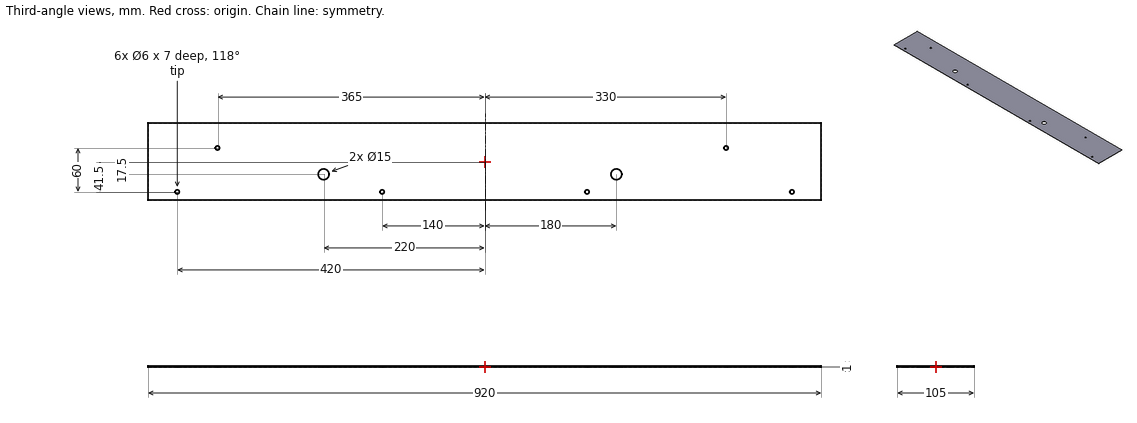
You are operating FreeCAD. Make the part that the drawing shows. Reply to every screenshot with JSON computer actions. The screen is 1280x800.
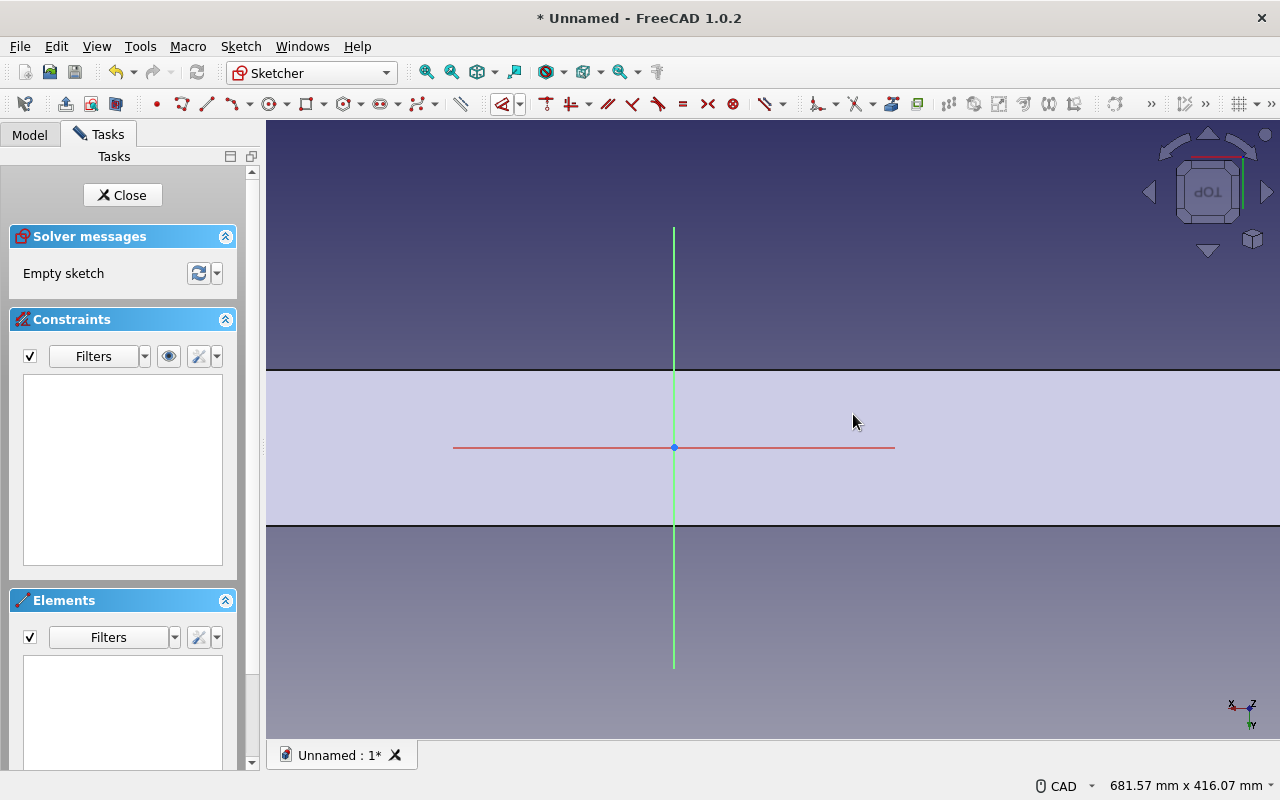
{"action": "left_click", "coordinate": [268, 104]}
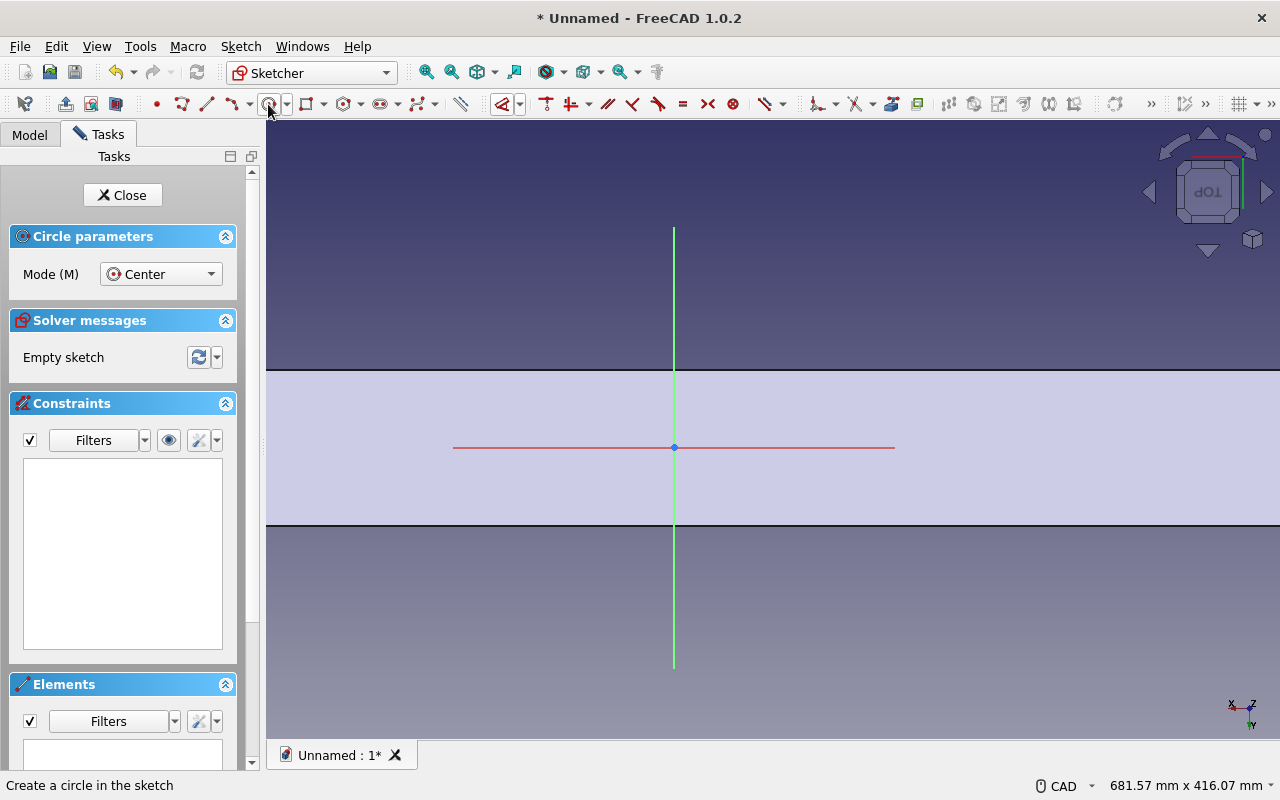
{"action": "scroll", "coordinate": [1002, 422], "scroll_direction": "up", "scroll_amount": 4}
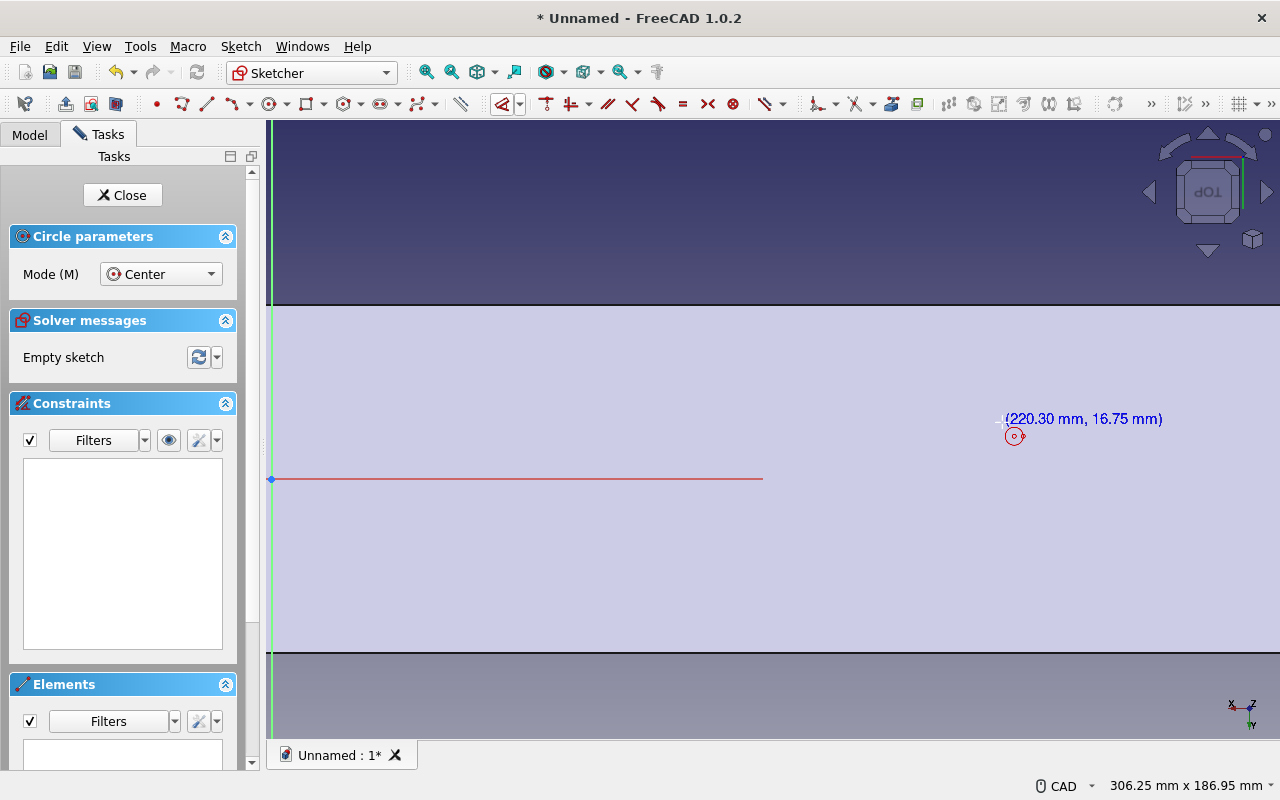
{"action": "left_click", "coordinate": [1000, 421]}
{"action": "left_click", "coordinate": [1018, 404]}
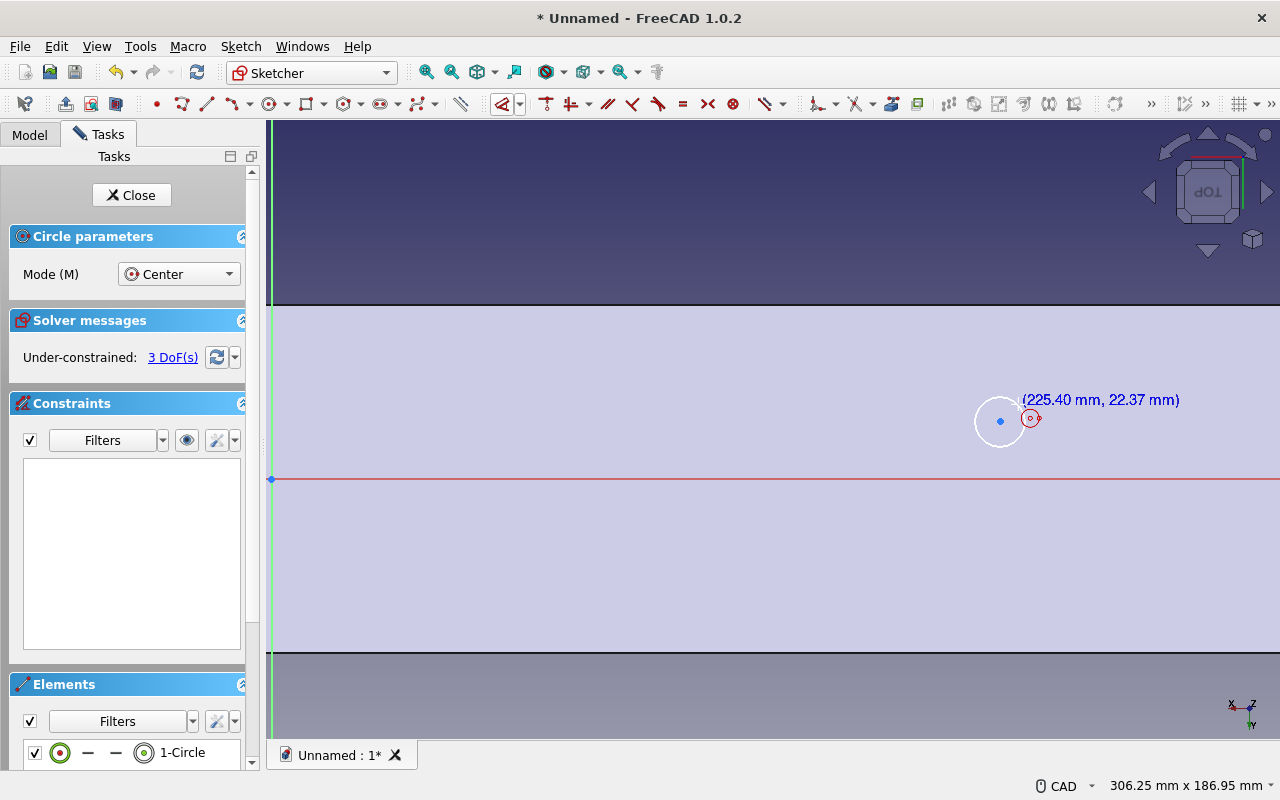
{"action": "scroll", "coordinate": [1004, 423], "scroll_direction": "down", "scroll_amount": 4}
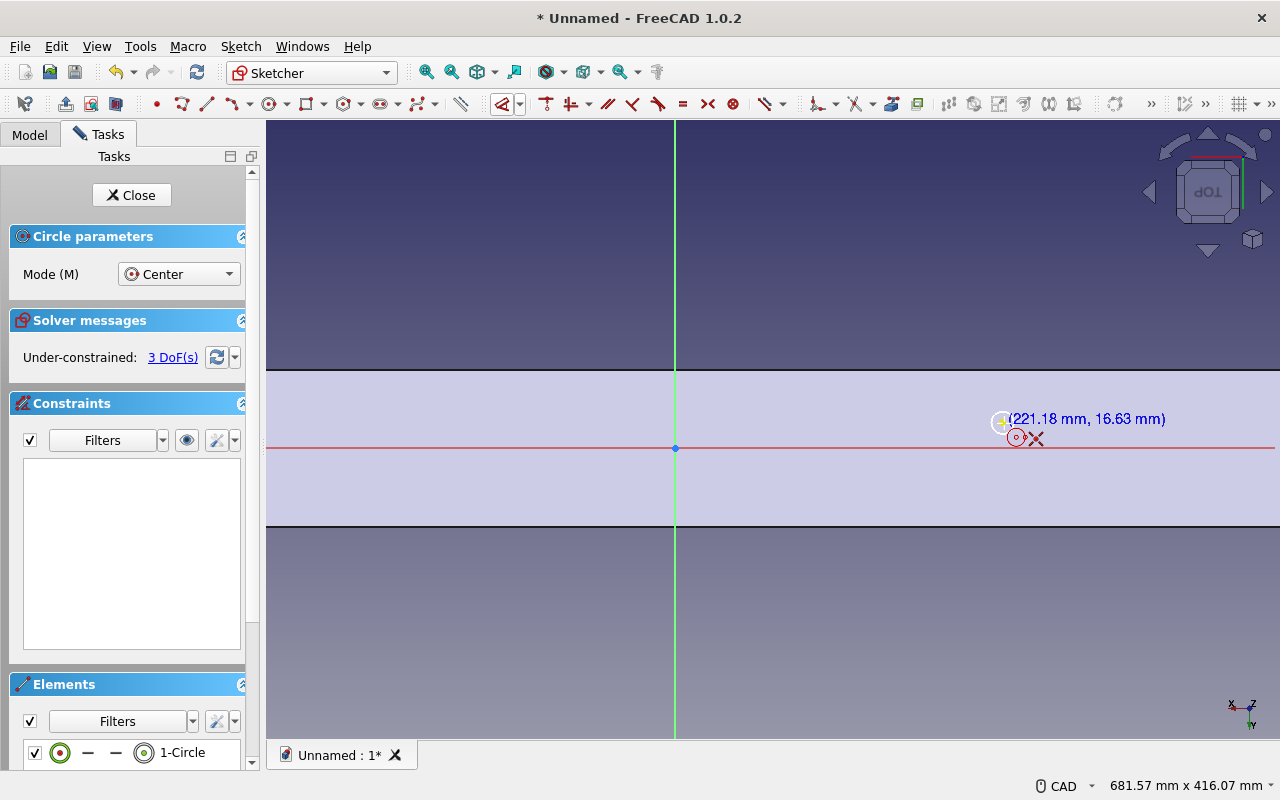
{"action": "scroll", "coordinate": [408, 422], "scroll_direction": "up", "scroll_amount": 4}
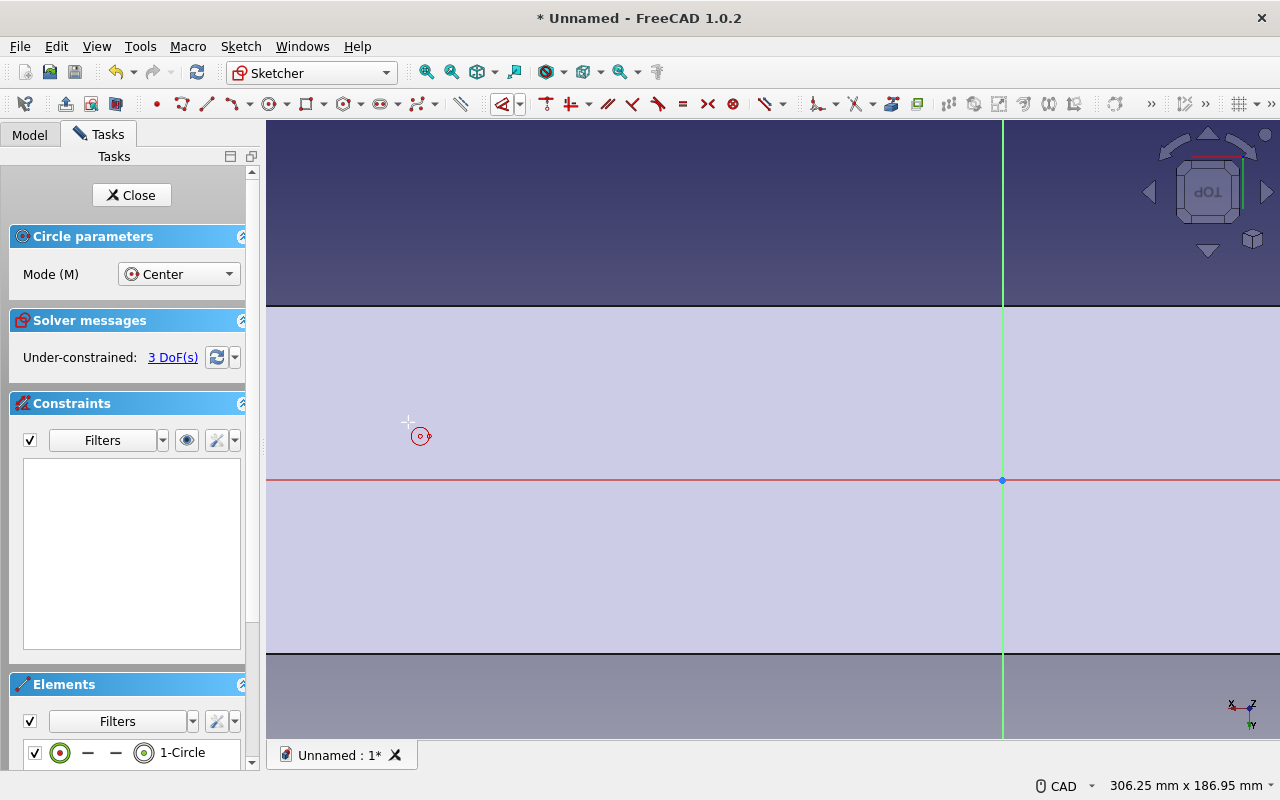
{"action": "left_click", "coordinate": [407, 422]}
{"action": "left_click", "coordinate": [424, 405]}
{"action": "key", "text": "Escape"}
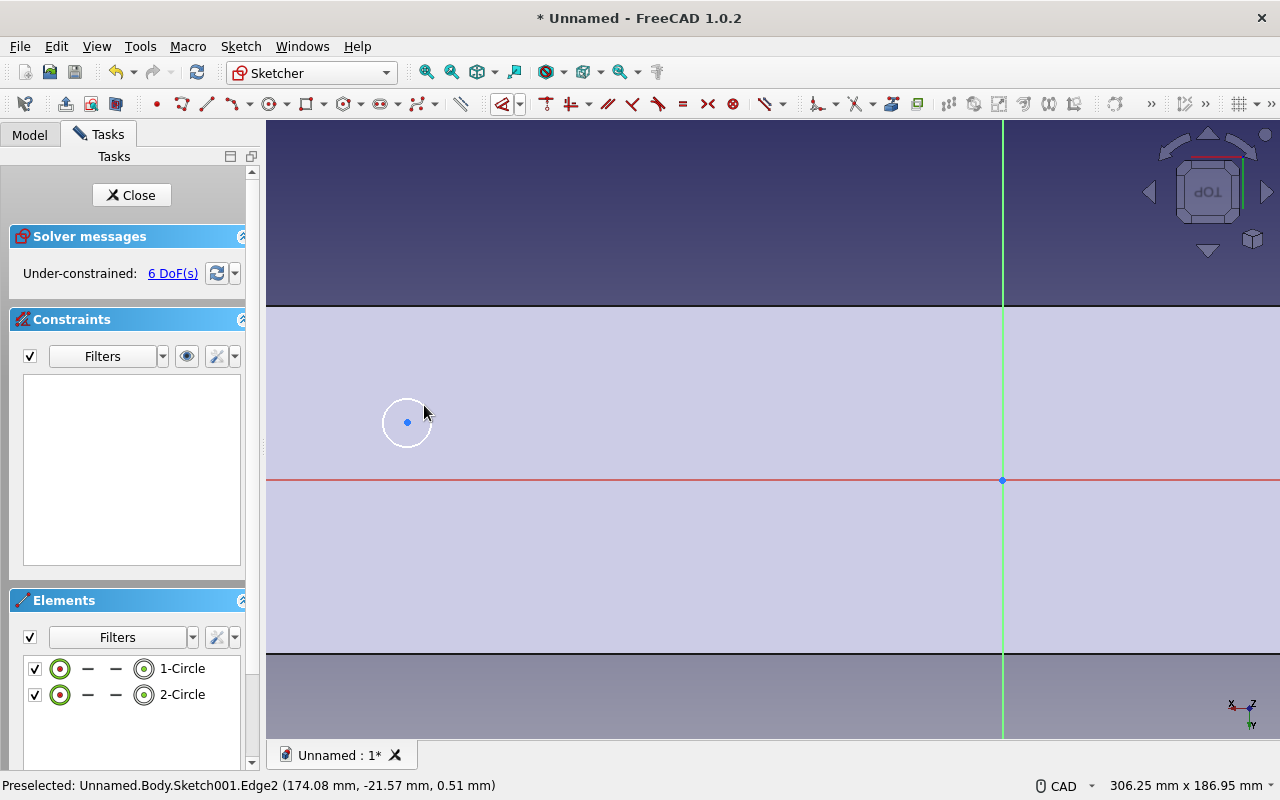
{"action": "scroll", "coordinate": [407, 422], "scroll_direction": "down", "scroll_amount": 4}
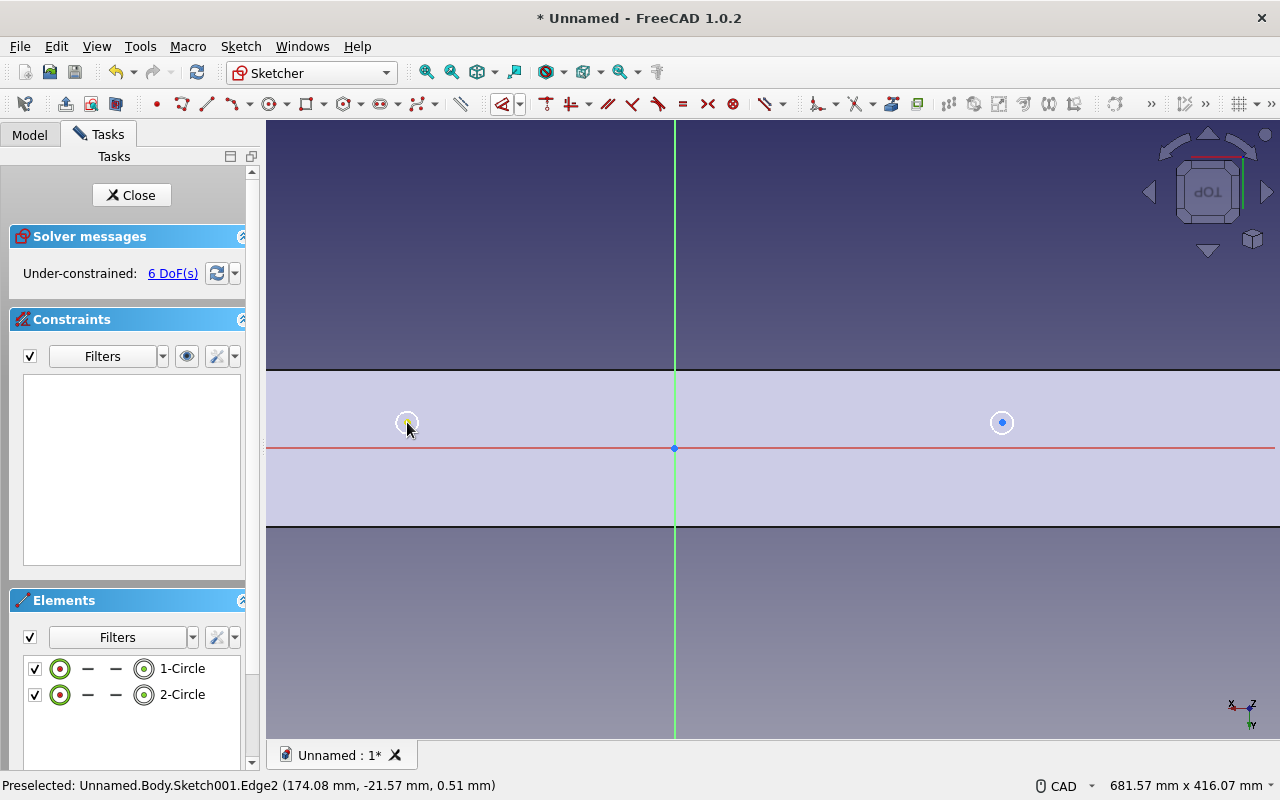
{"action": "scroll", "coordinate": [1010, 415], "scroll_direction": "up", "scroll_amount": 2}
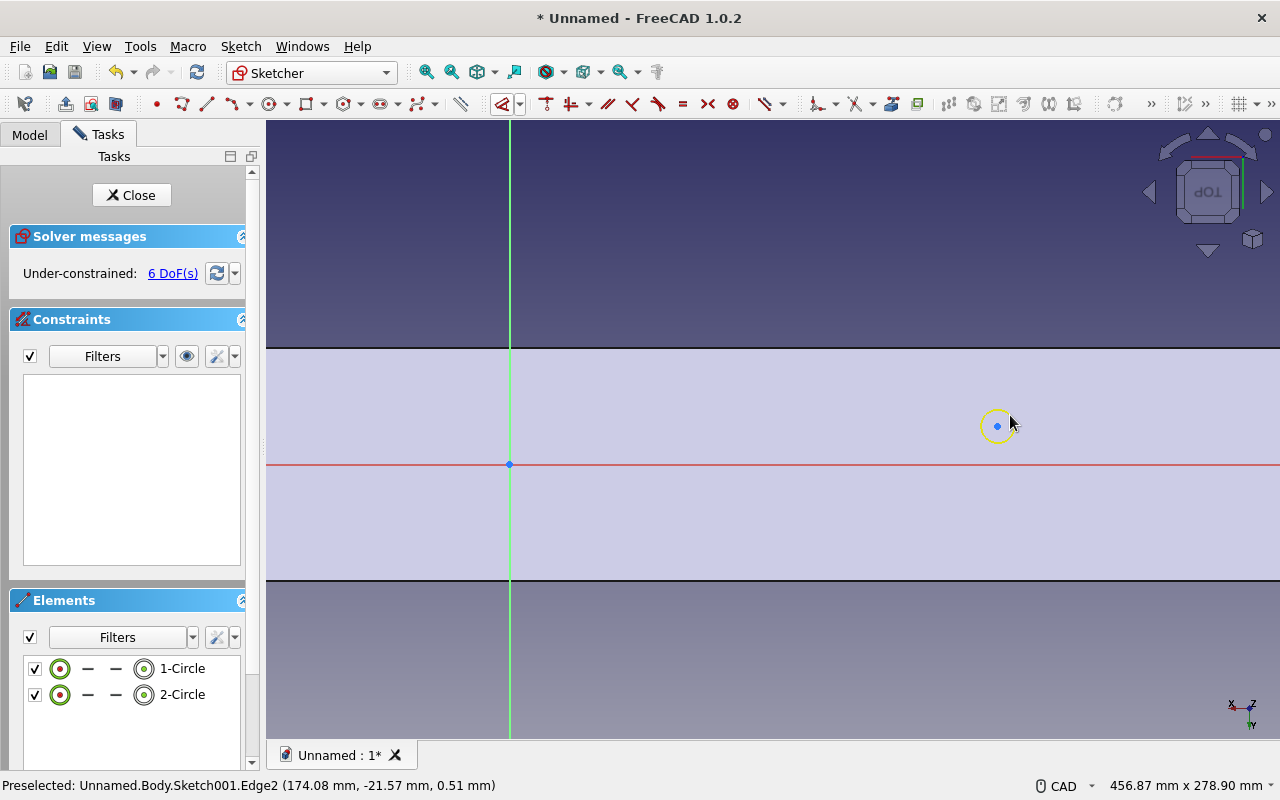
{"action": "left_click", "coordinate": [1009, 415]}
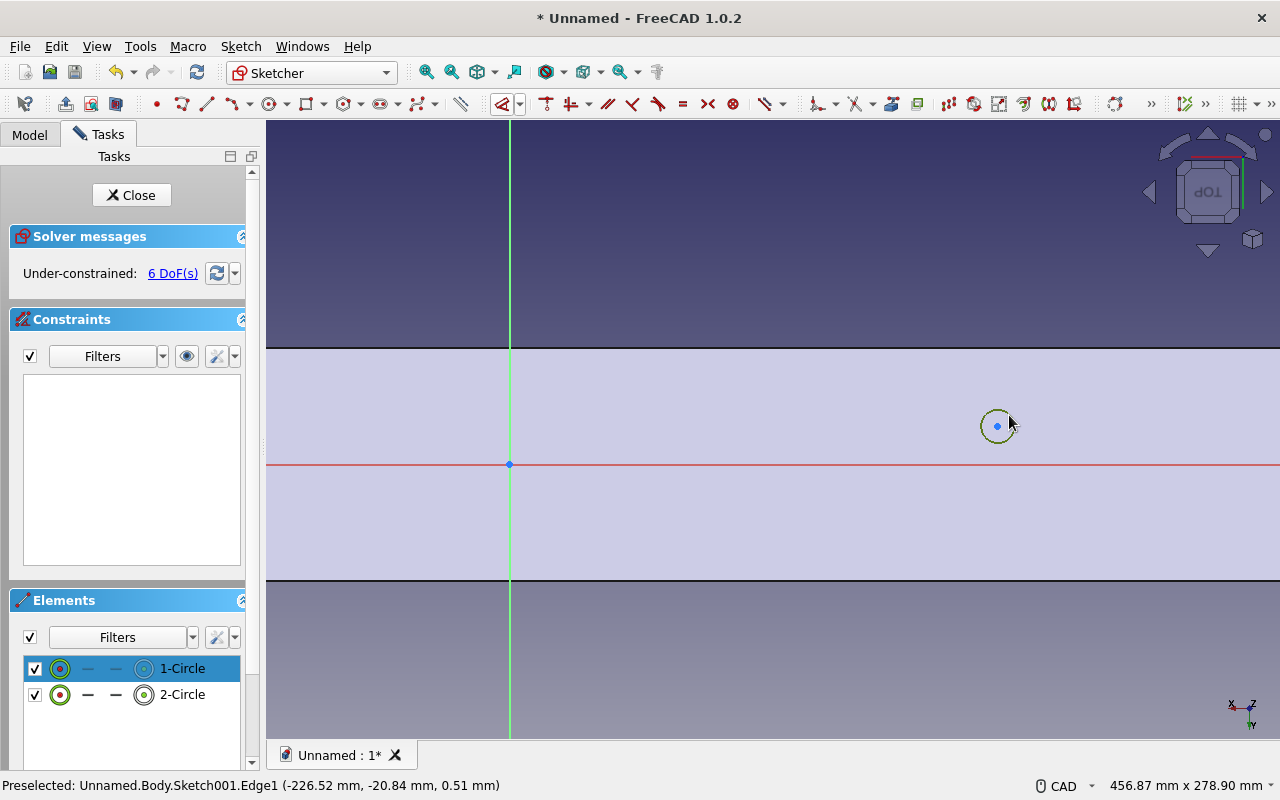
{"action": "scroll", "coordinate": [1011, 414], "scroll_direction": "down", "scroll_amount": 2}